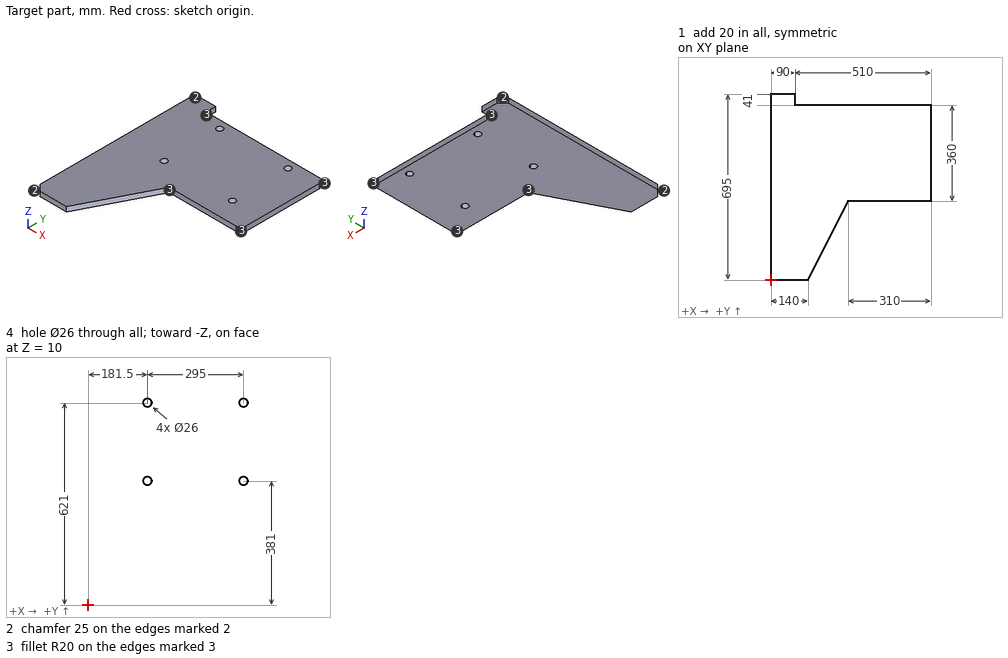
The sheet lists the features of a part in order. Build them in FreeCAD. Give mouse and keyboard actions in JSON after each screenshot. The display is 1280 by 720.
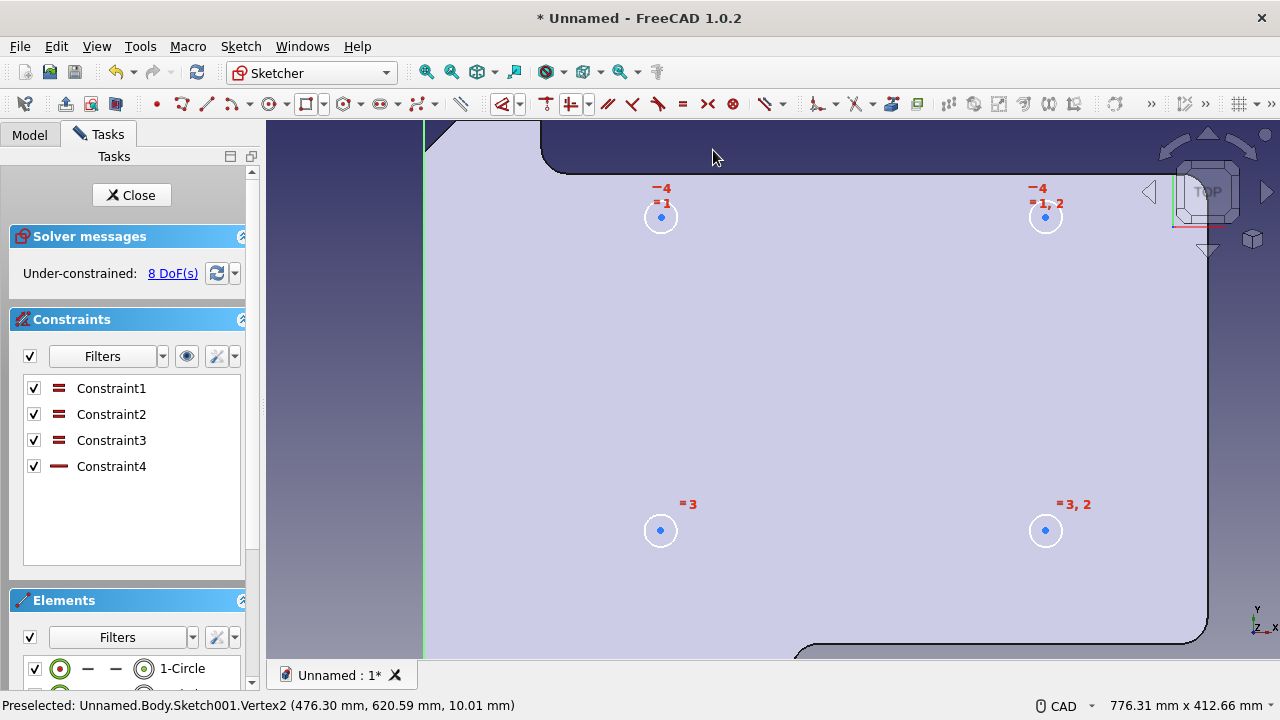
{"action": "left_click", "coordinate": [1046, 217]}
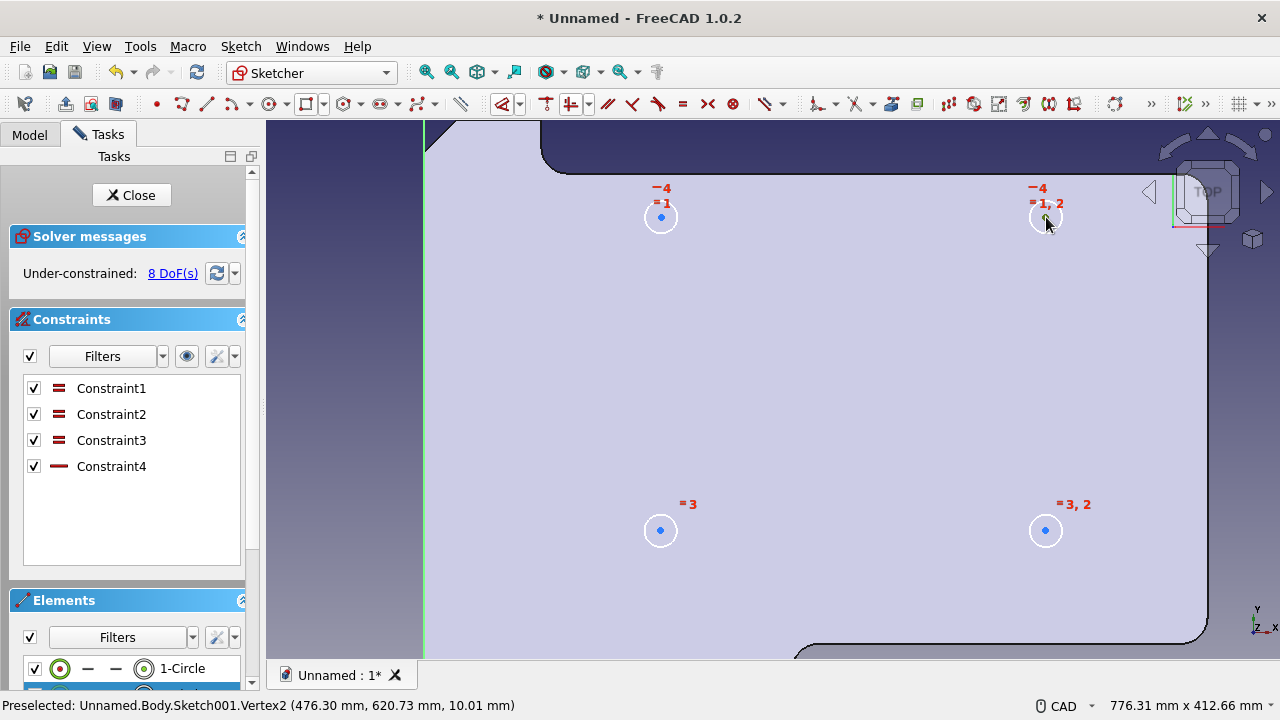
{"action": "left_click", "coordinate": [1046, 531]}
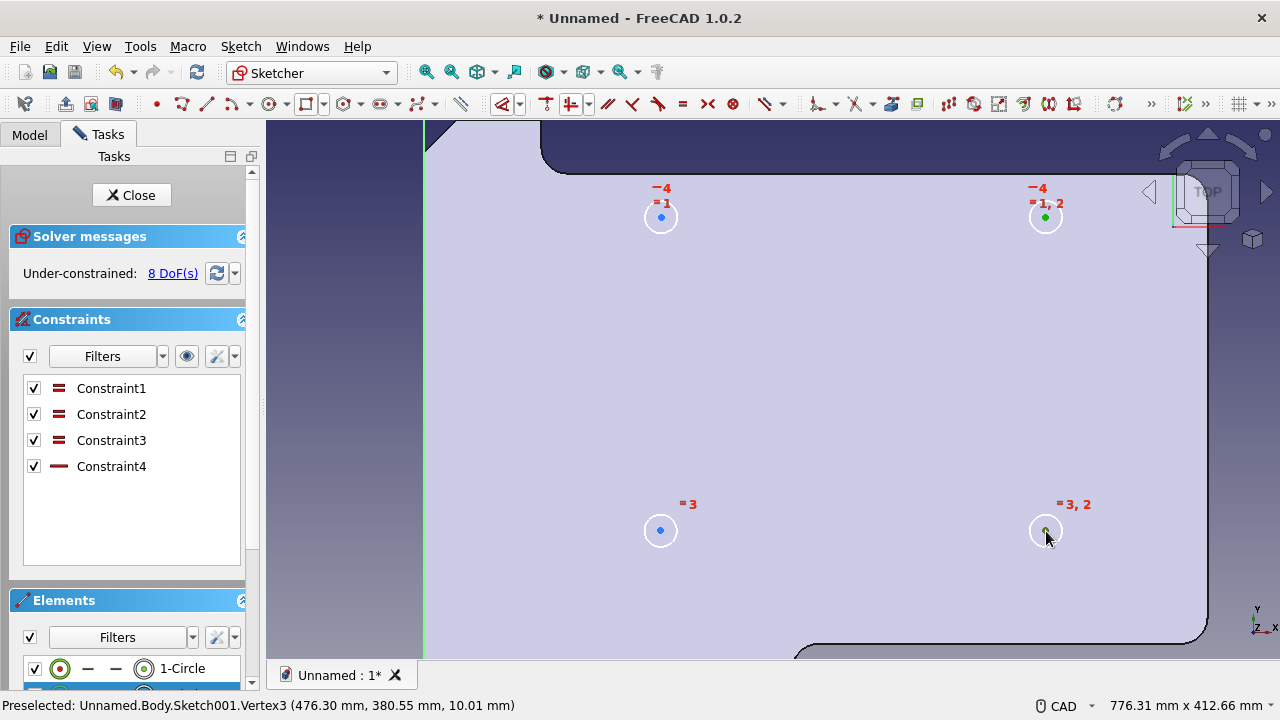
{"action": "left_click", "coordinate": [588, 104]}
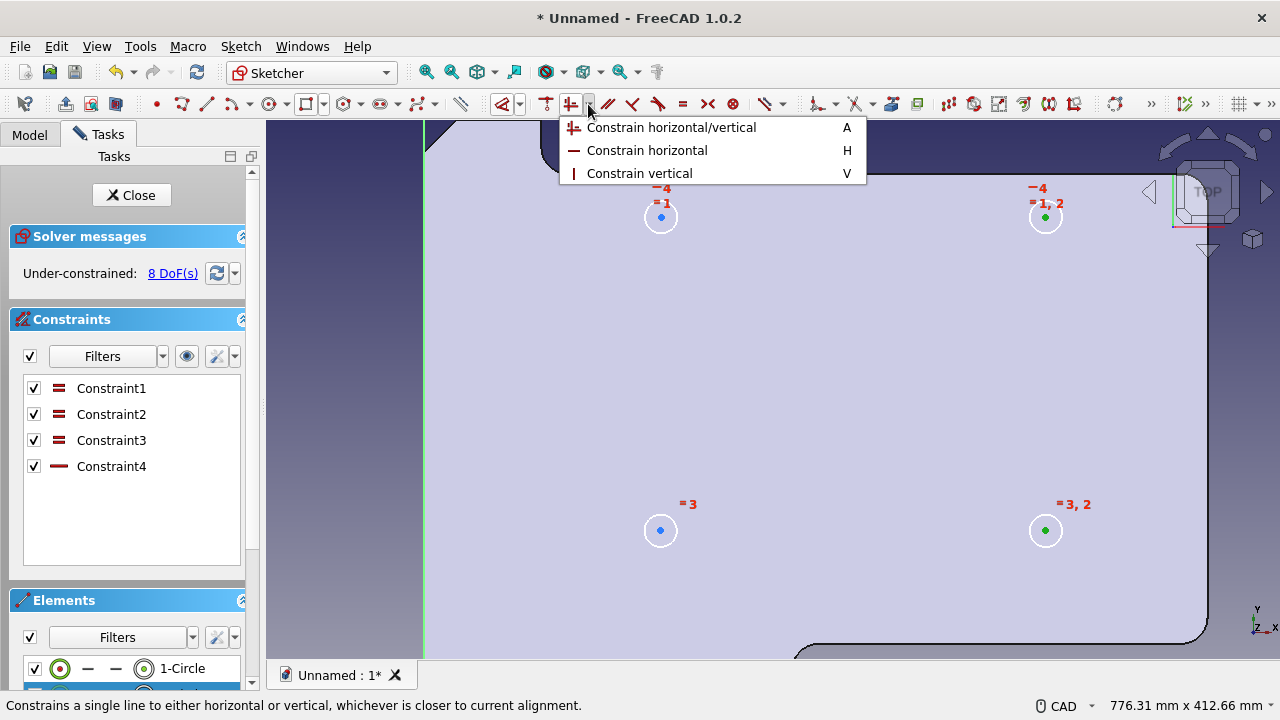
{"action": "left_click", "coordinate": [713, 174]}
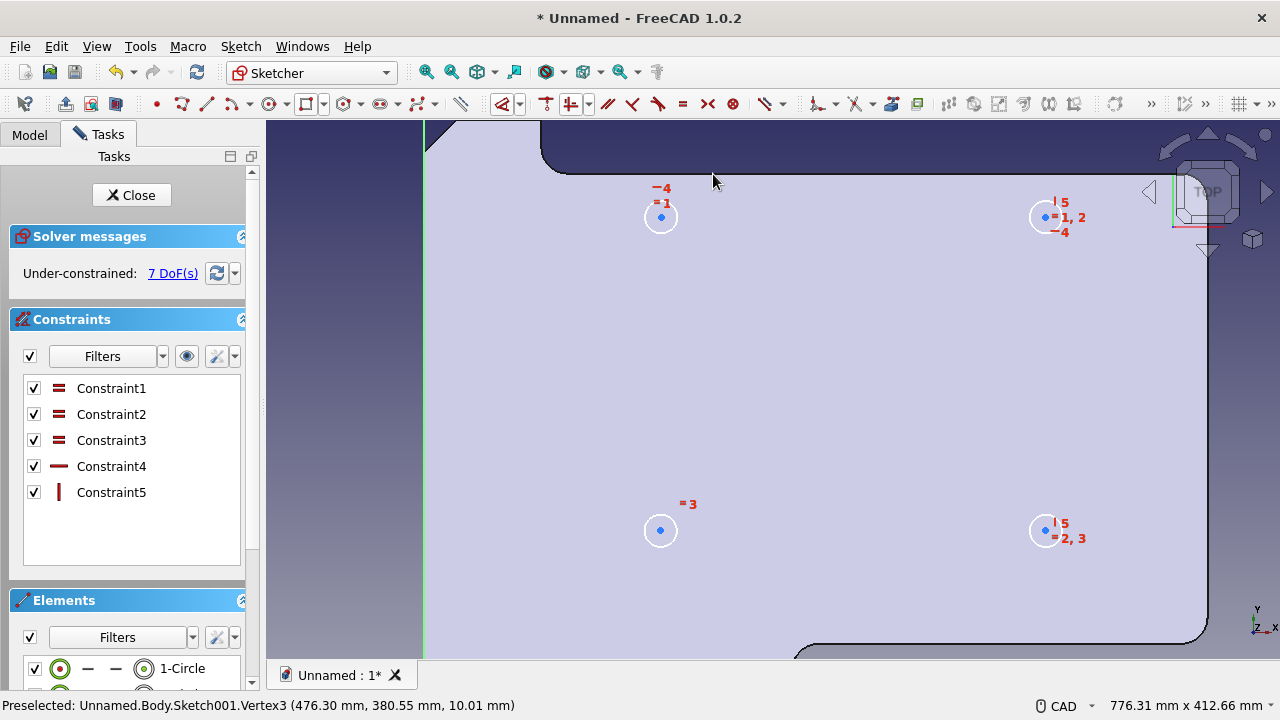
{"action": "left_click", "coordinate": [661, 217]}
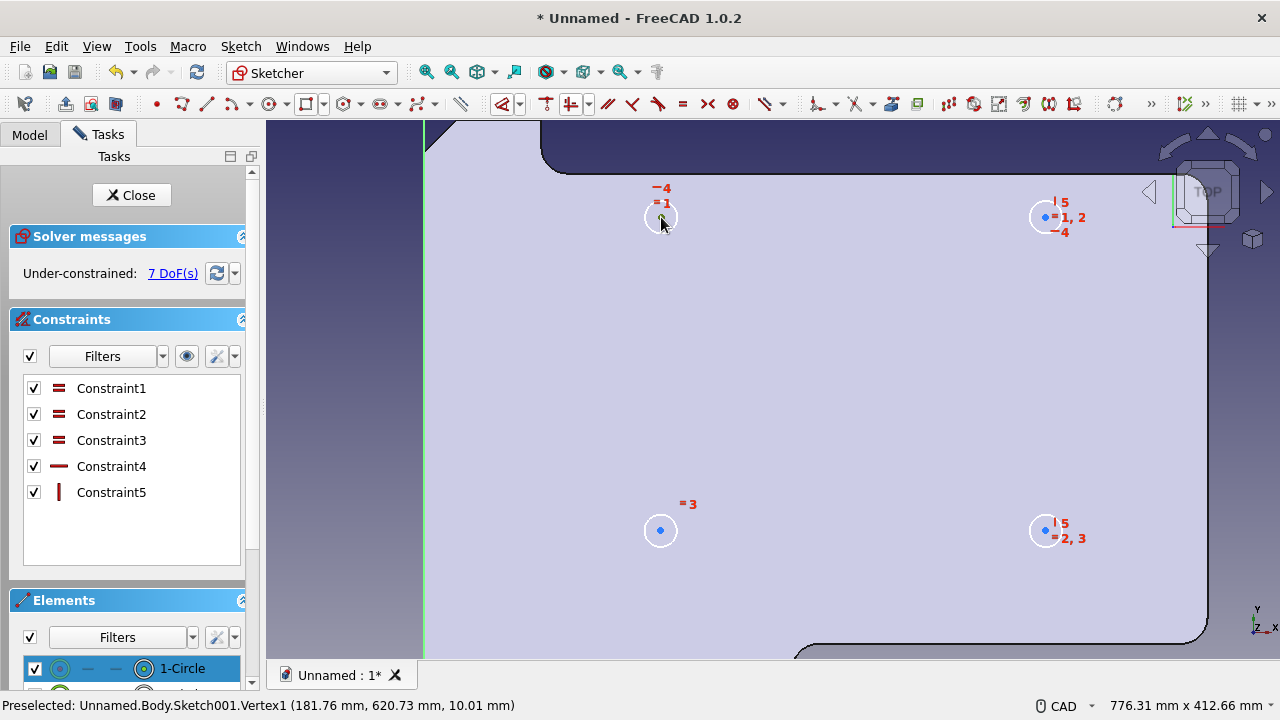
{"action": "left_click", "coordinate": [661, 531]}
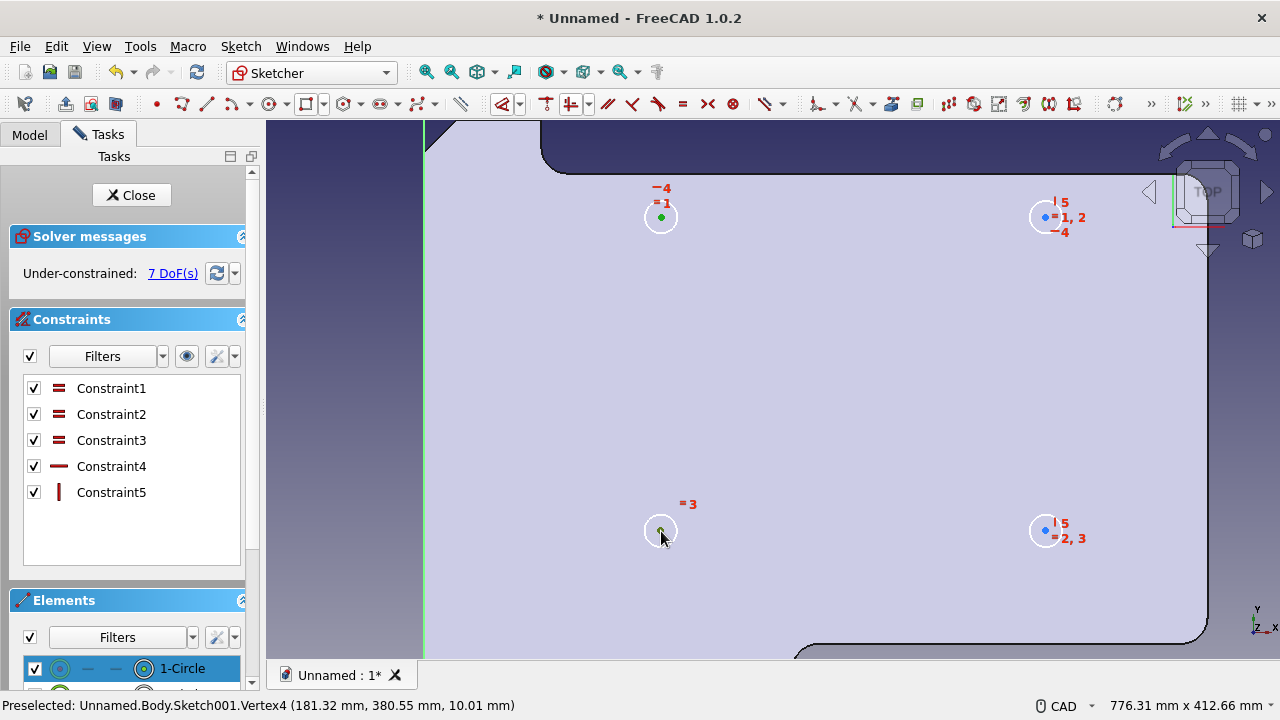
{"action": "left_click", "coordinate": [588, 104]}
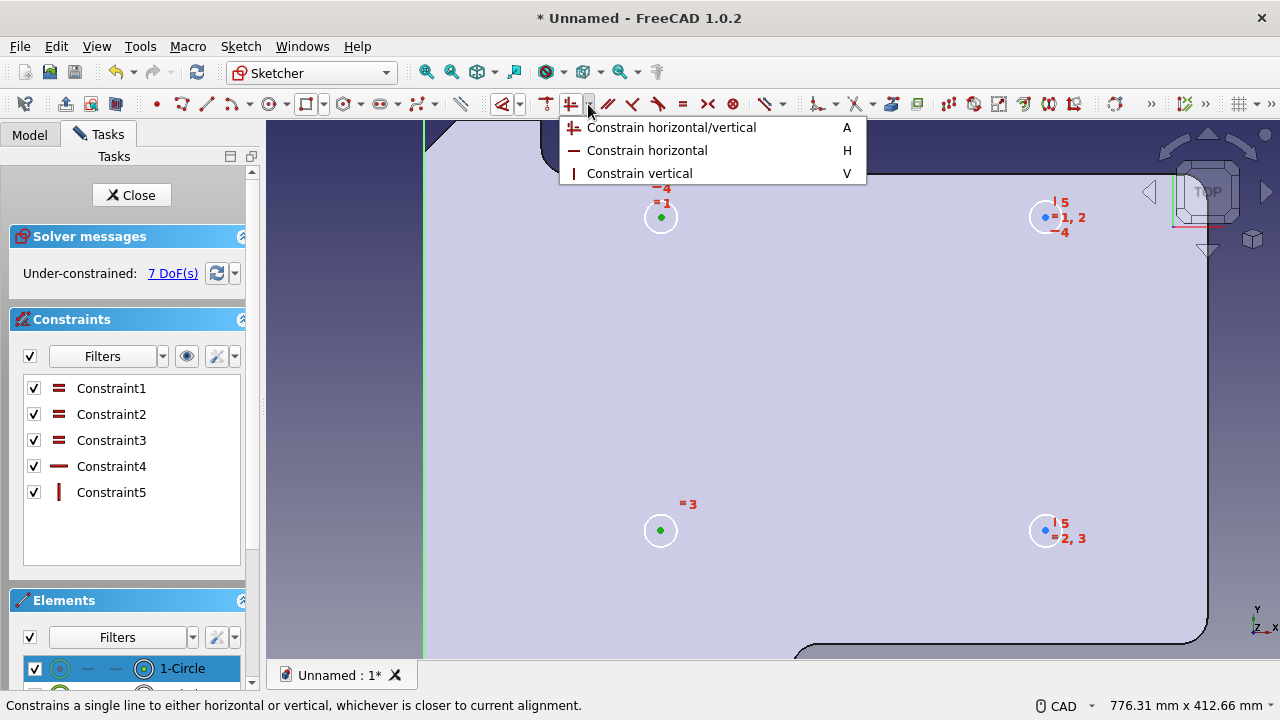
{"action": "left_click", "coordinate": [713, 174]}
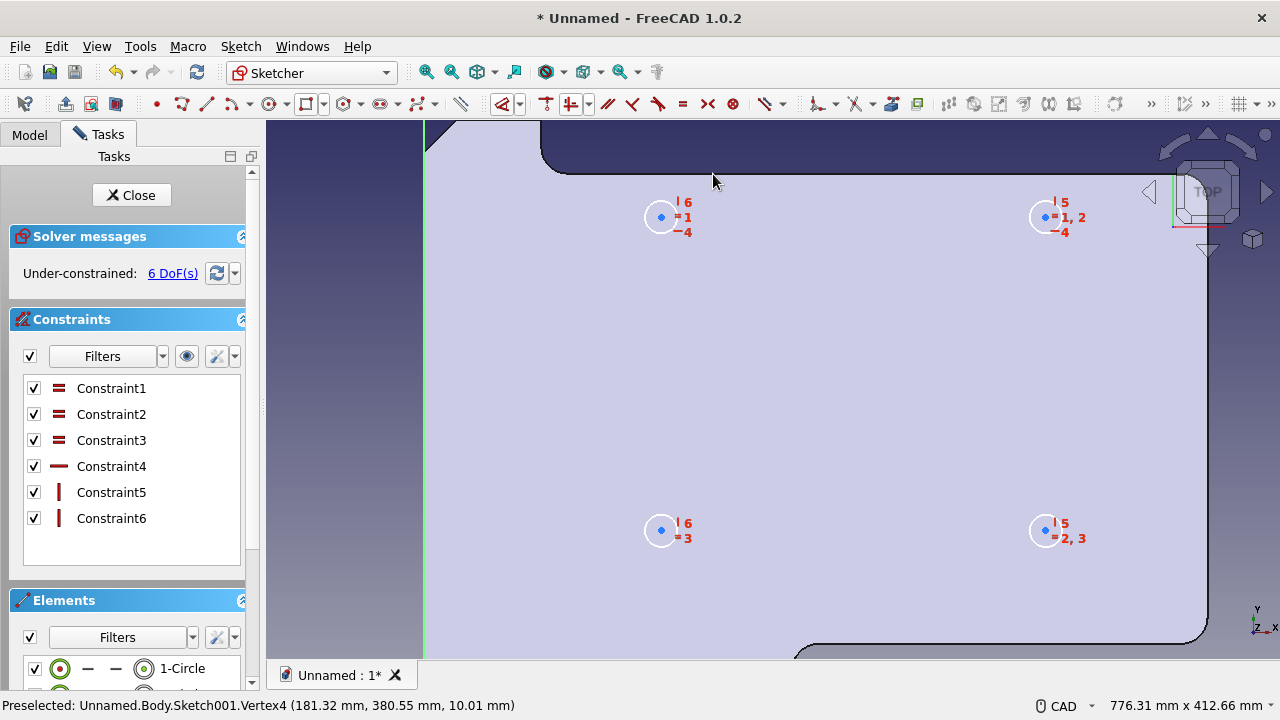
{"action": "left_click", "coordinate": [1046, 531]}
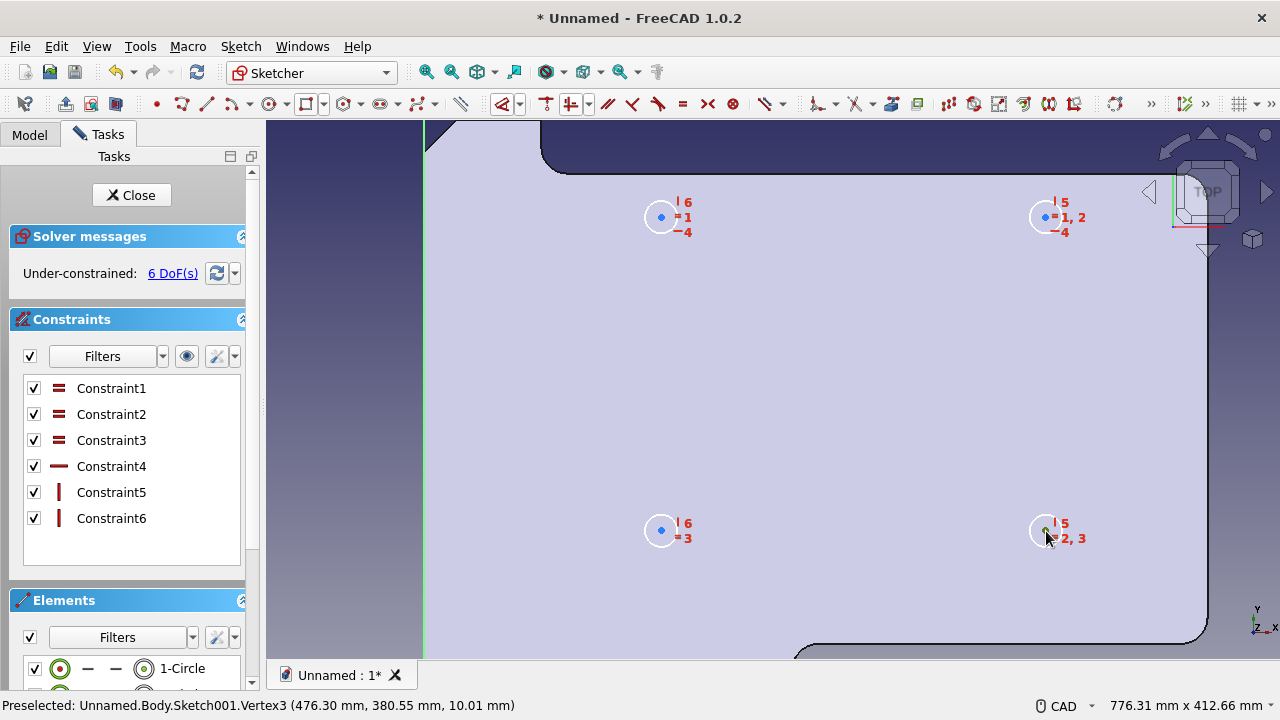
{"action": "left_click", "coordinate": [661, 531]}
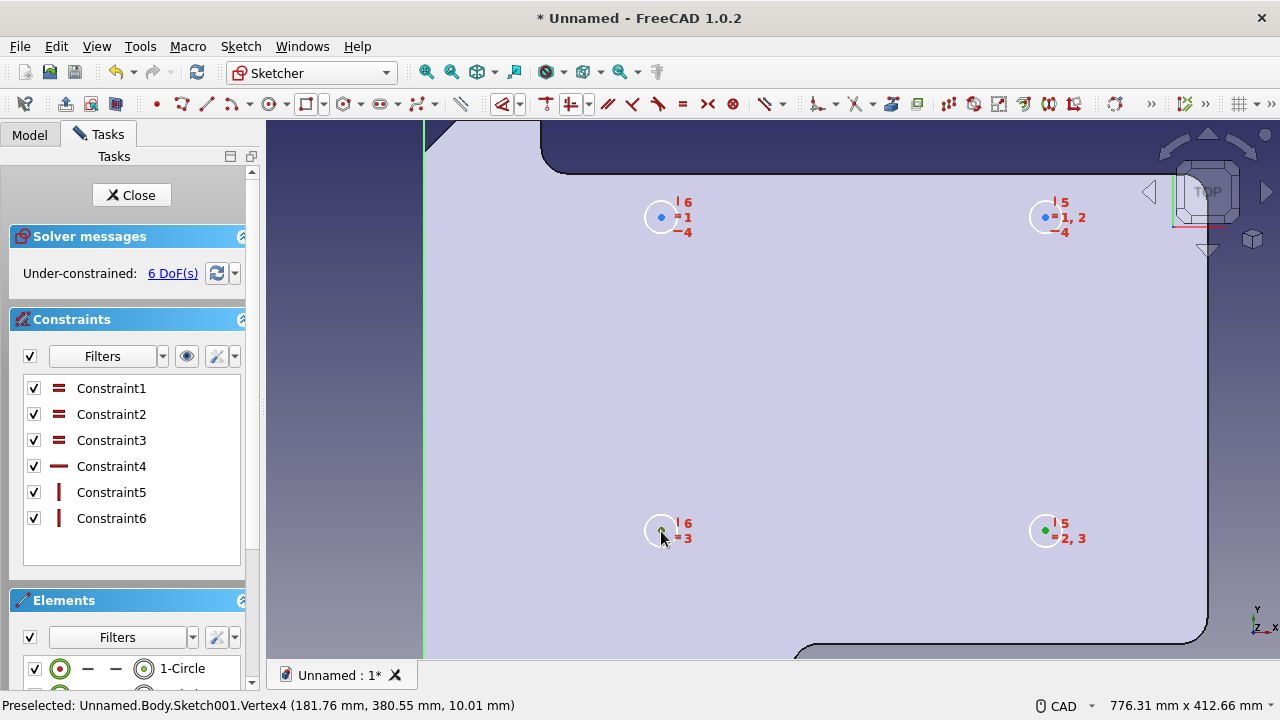
{"action": "key", "text": "h"}